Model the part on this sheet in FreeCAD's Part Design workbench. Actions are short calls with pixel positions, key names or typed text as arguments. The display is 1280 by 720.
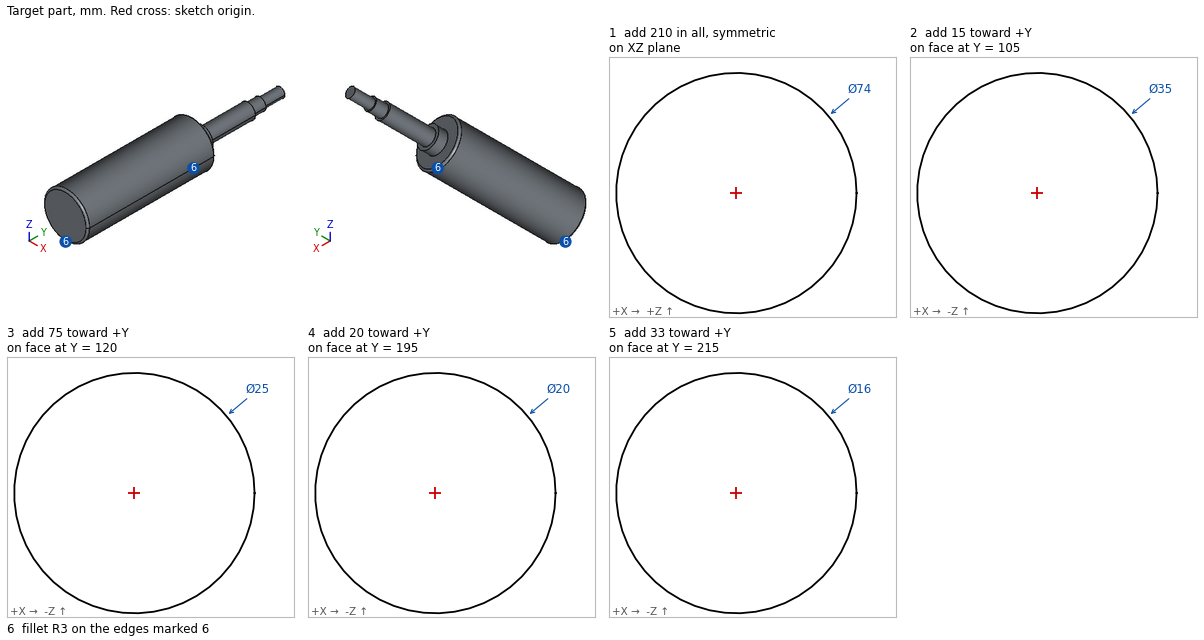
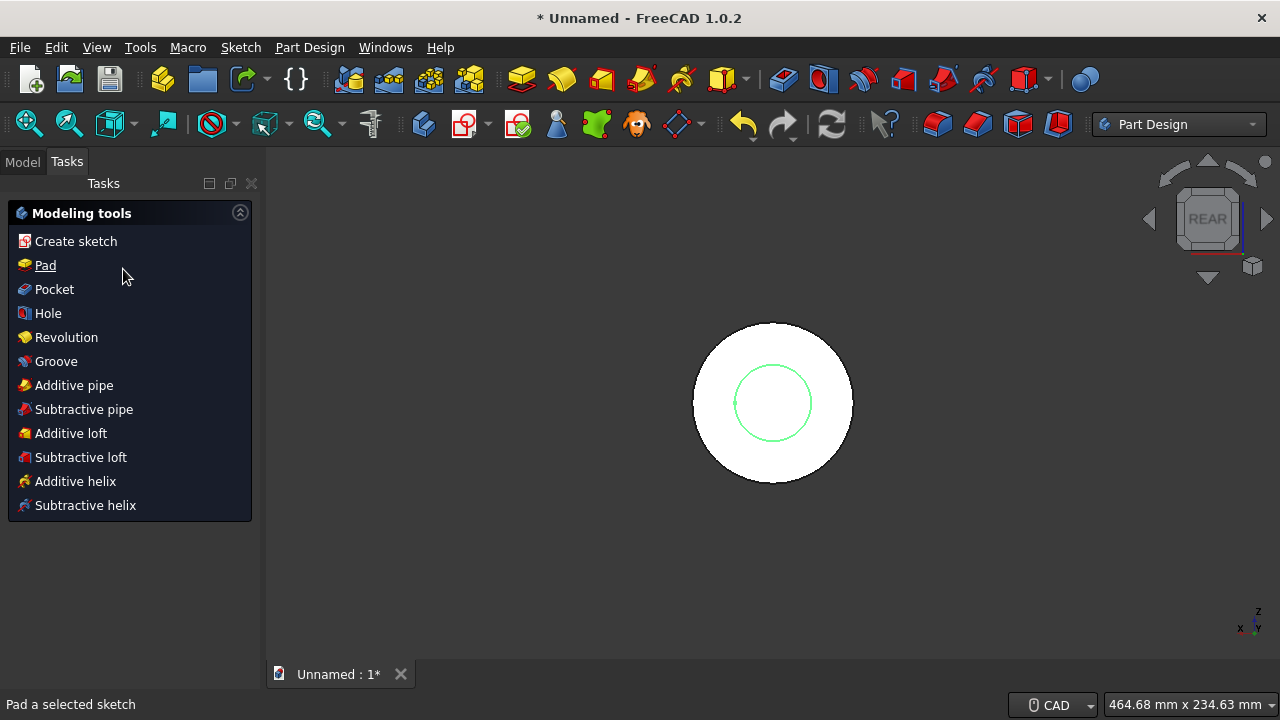
click(522, 80)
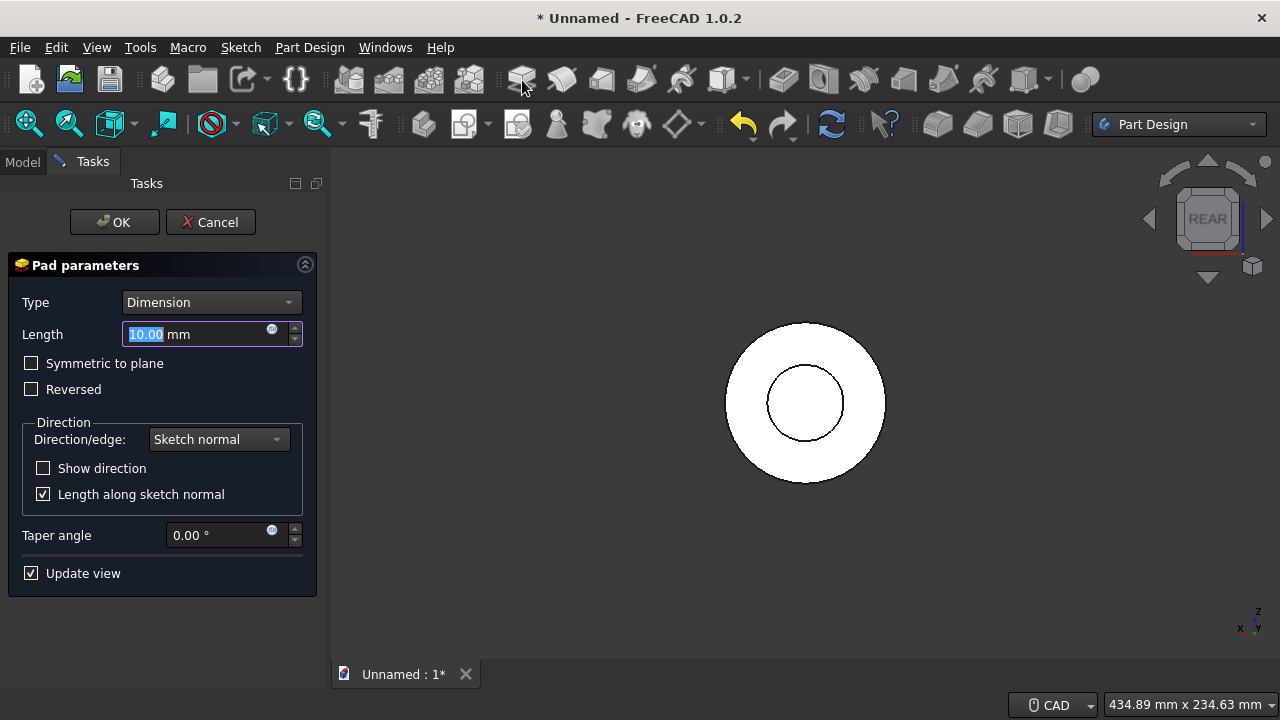
text(15)
key(Tab)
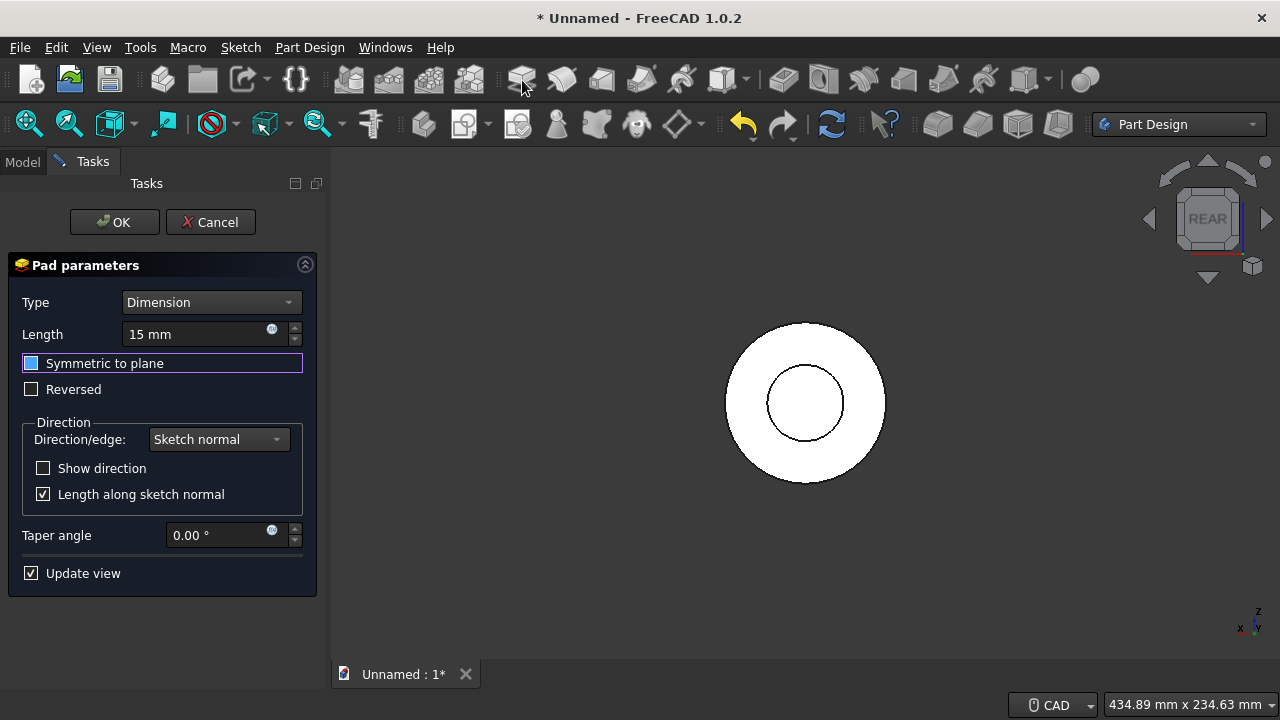
click(115, 222)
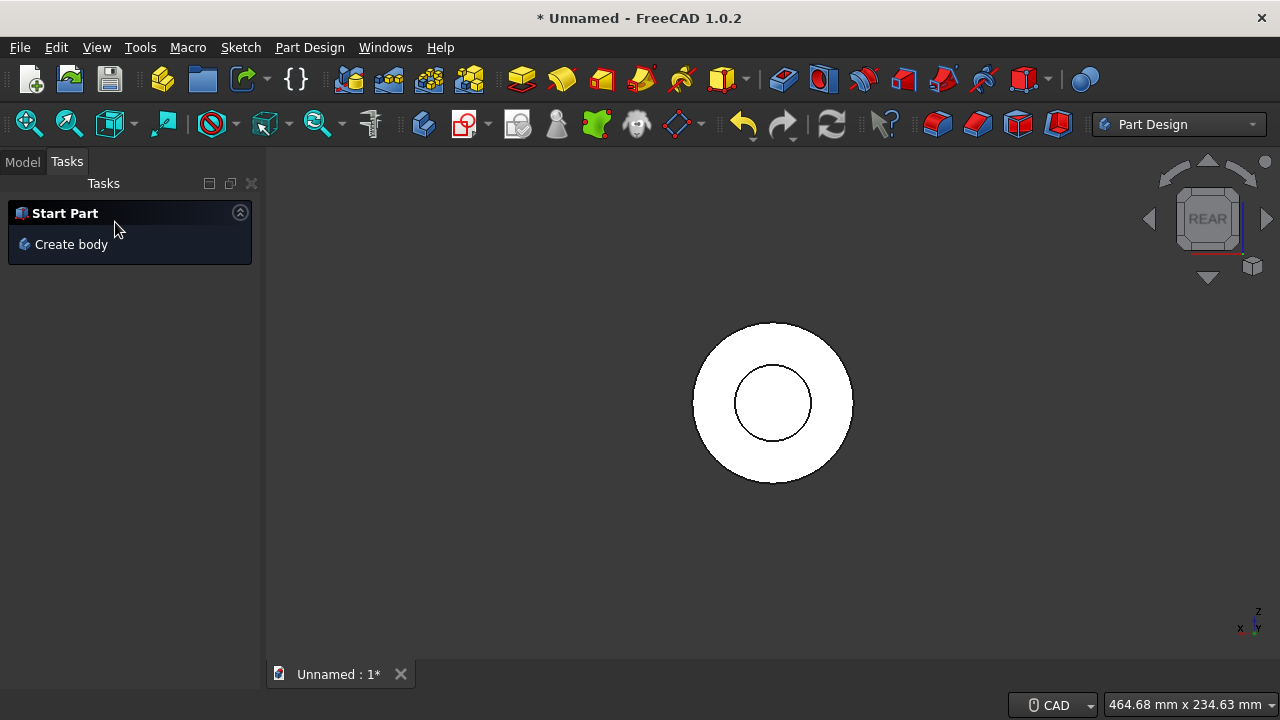
click(30, 124)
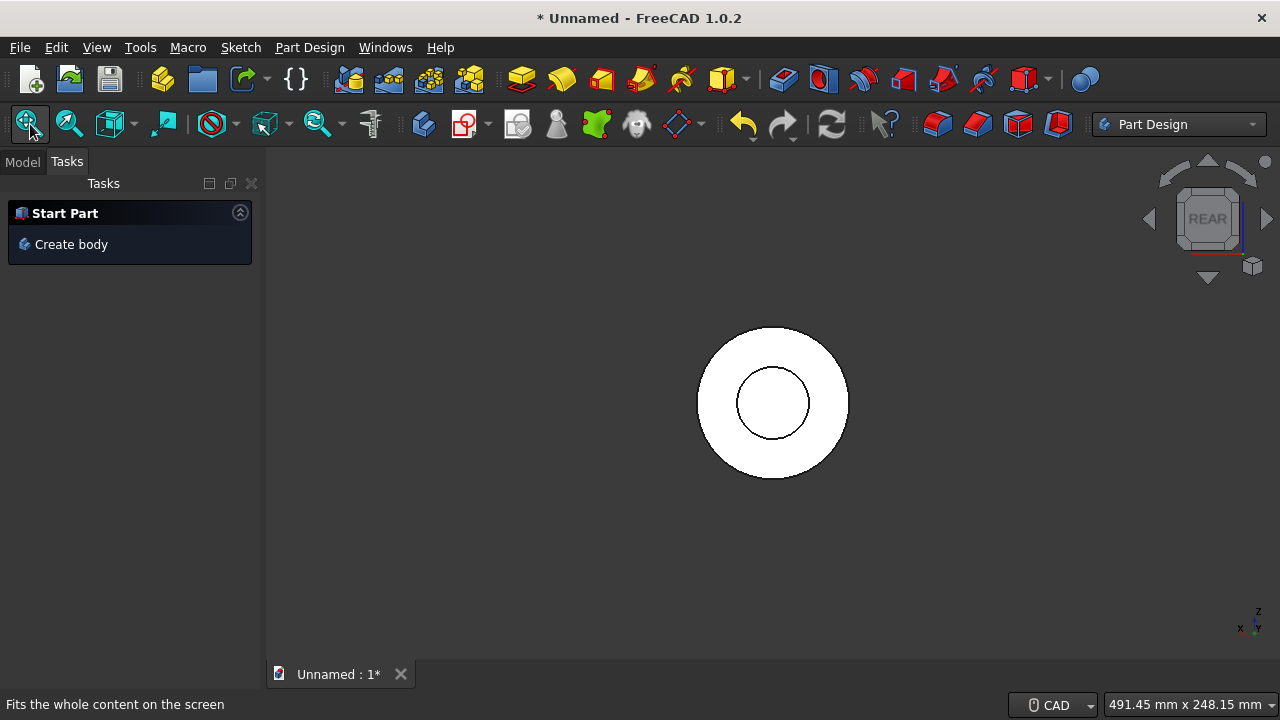
click(773, 402)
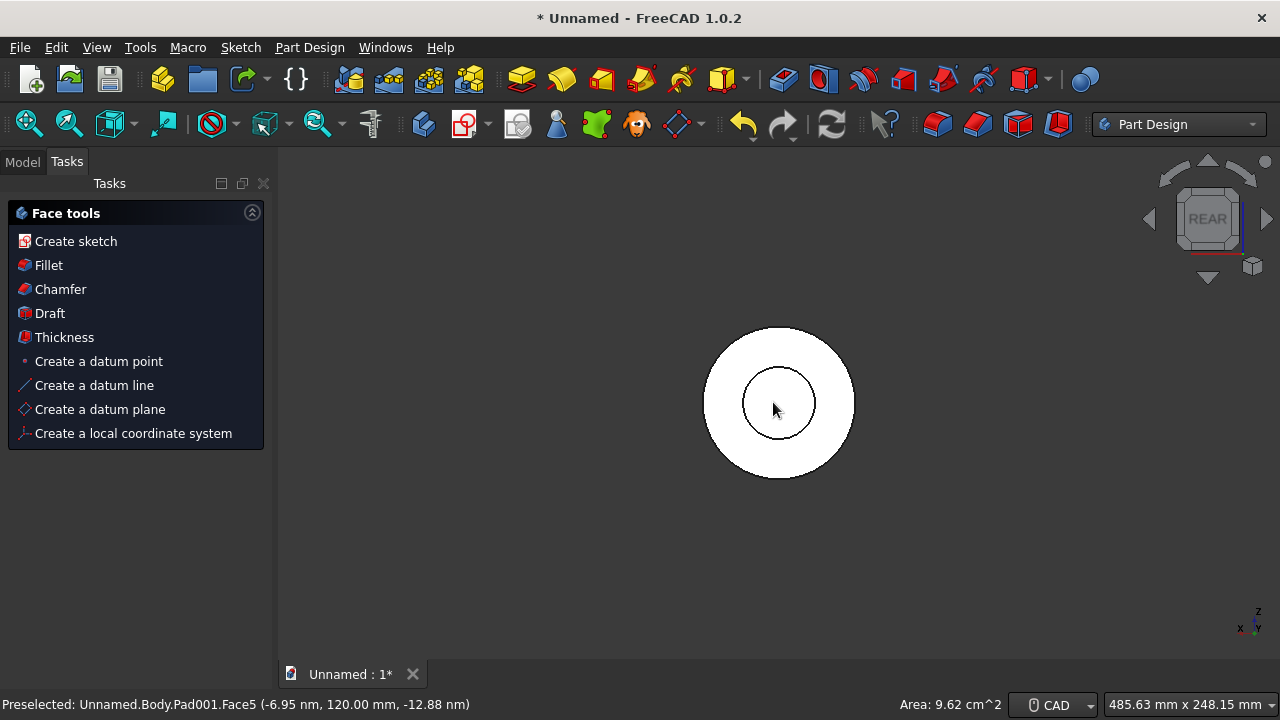
click(464, 124)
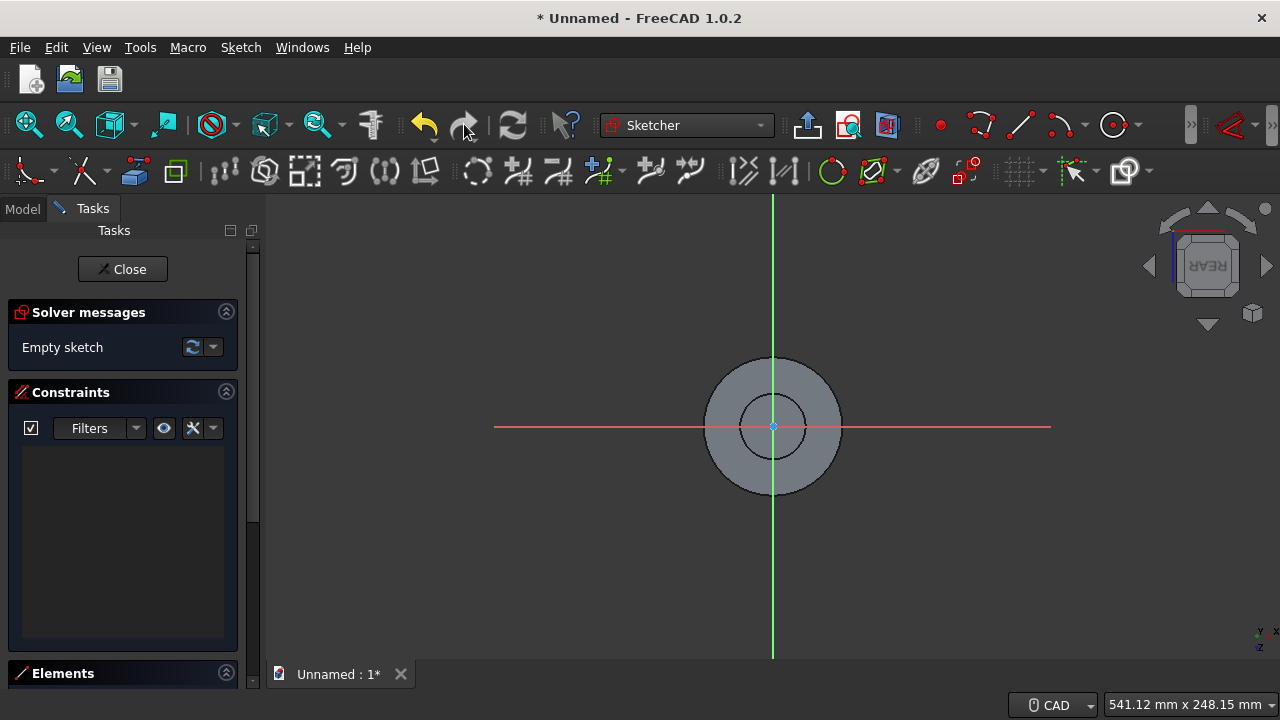
scroll(787, 426, up, 9)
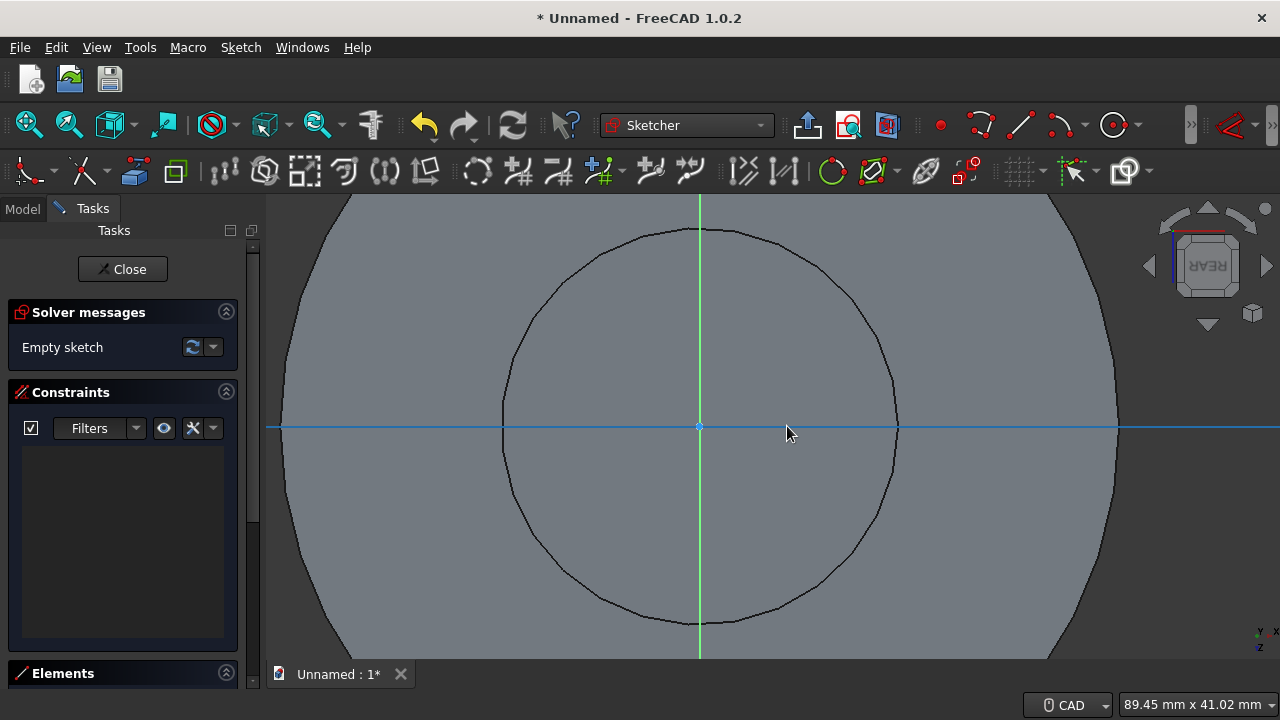
click(1114, 126)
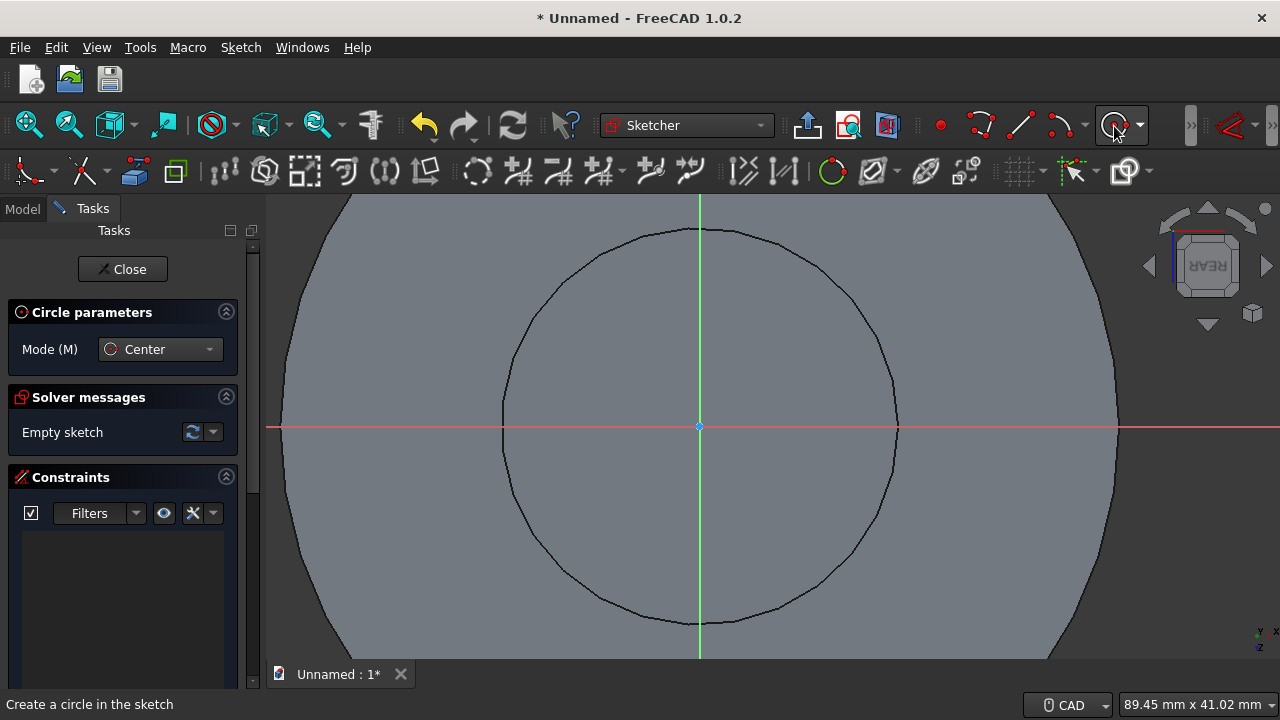
click(700, 426)
move(800, 326)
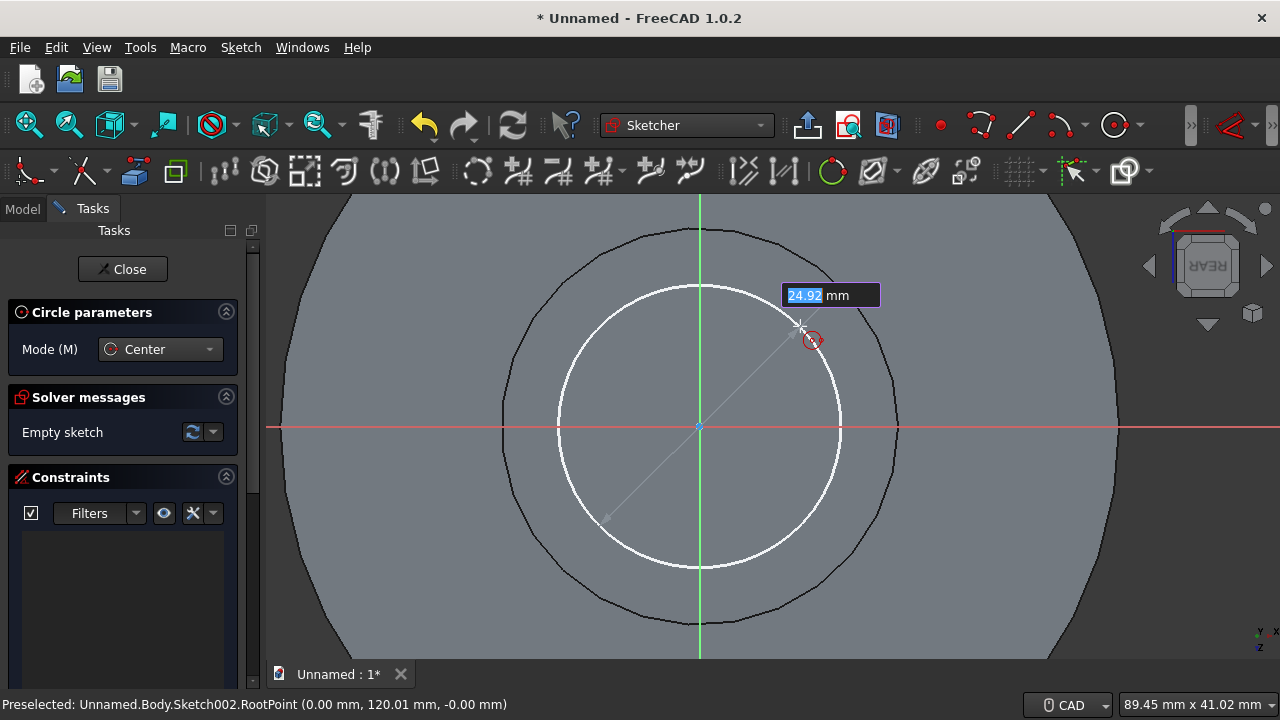
text(25)
key(Return)
key(Escape)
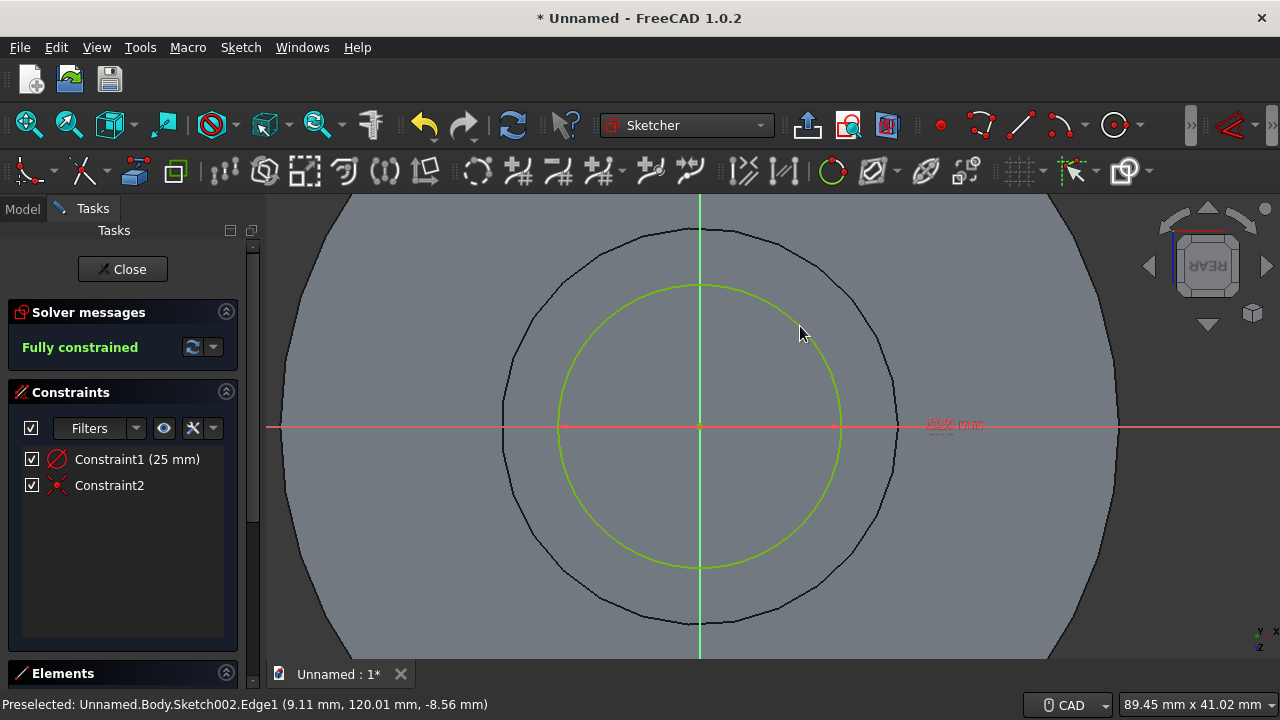
click(123, 269)